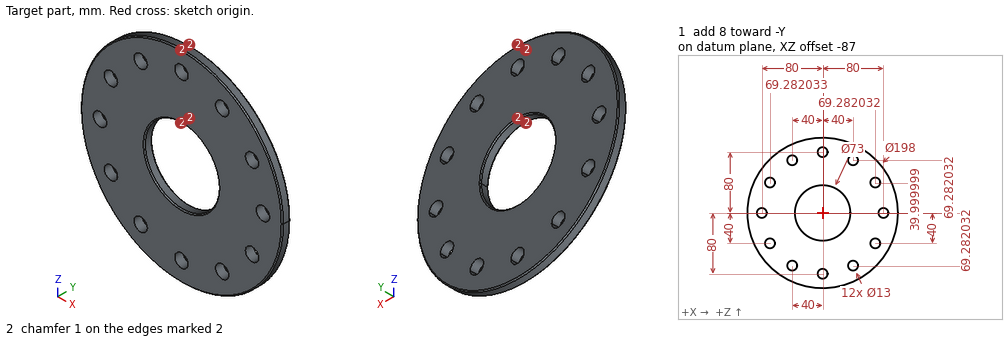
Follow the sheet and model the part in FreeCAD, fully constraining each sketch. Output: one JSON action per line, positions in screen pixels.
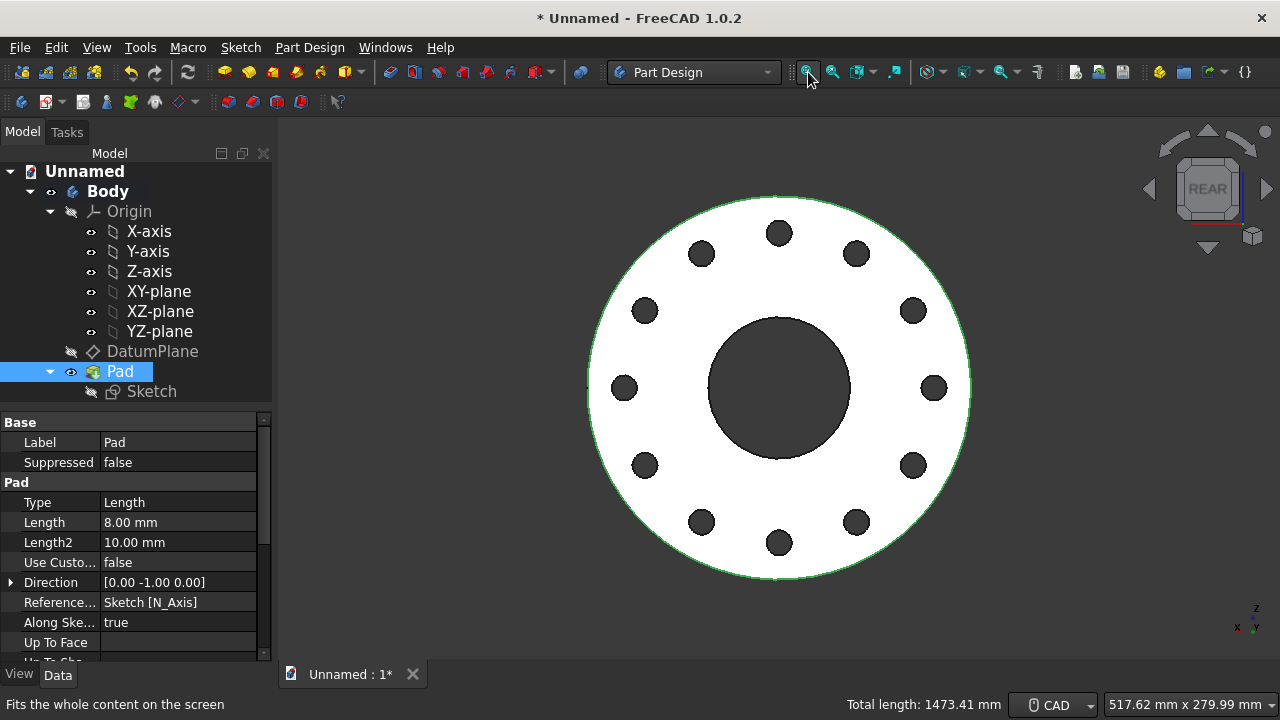
{"action": "left_click", "coordinate": [850, 387], "text": "ctrl"}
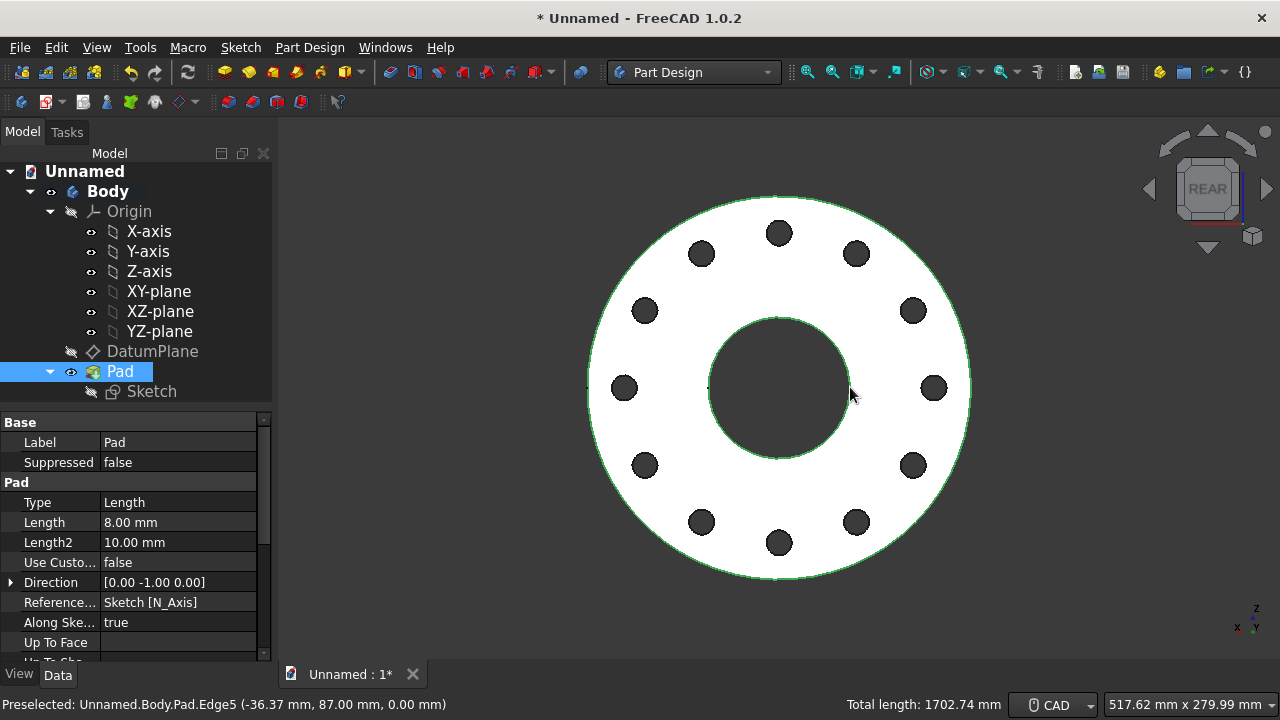
{"action": "left_click", "coordinate": [254, 102]}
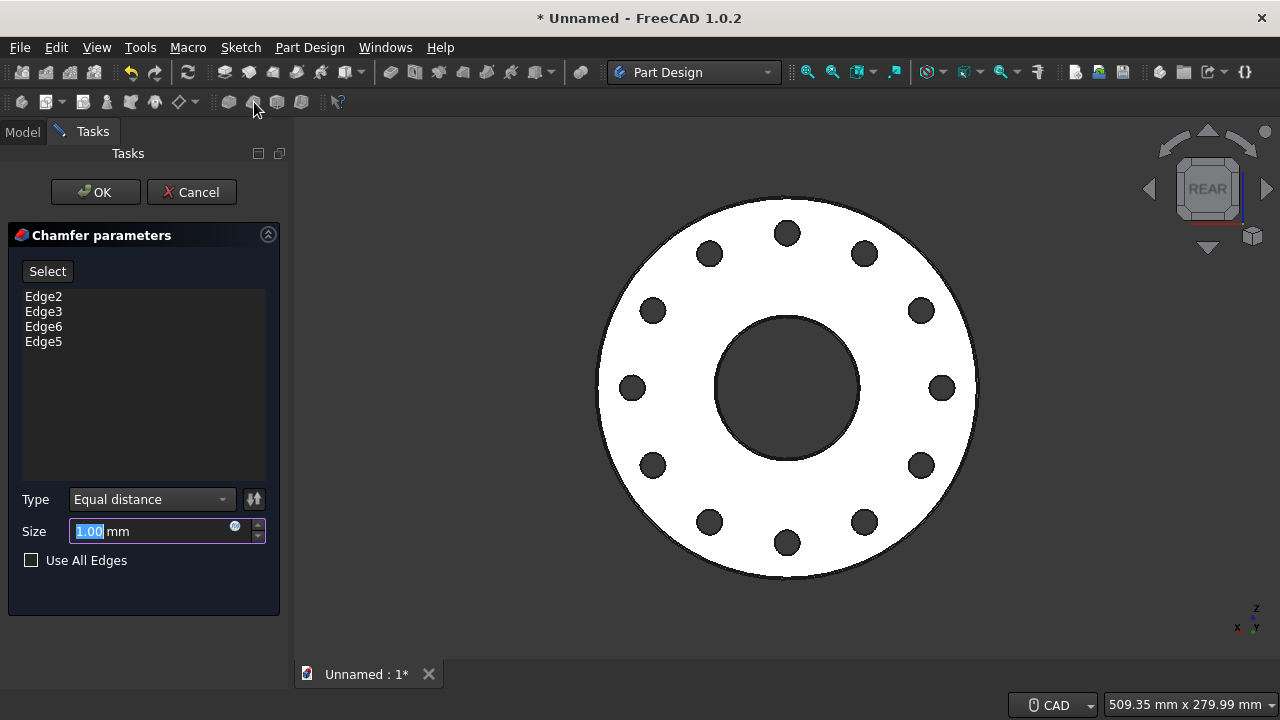
{"action": "type", "text": "1"}
{"action": "key", "text": "Tab"}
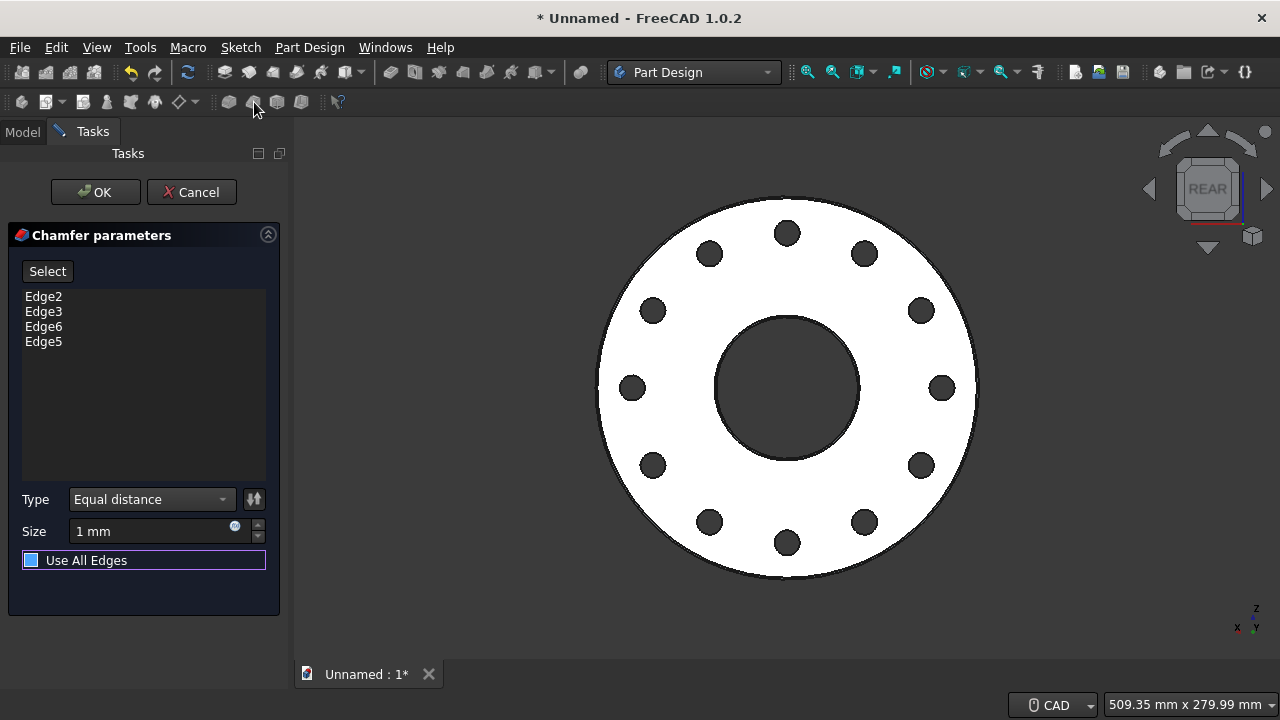
{"action": "left_click", "coordinate": [96, 192]}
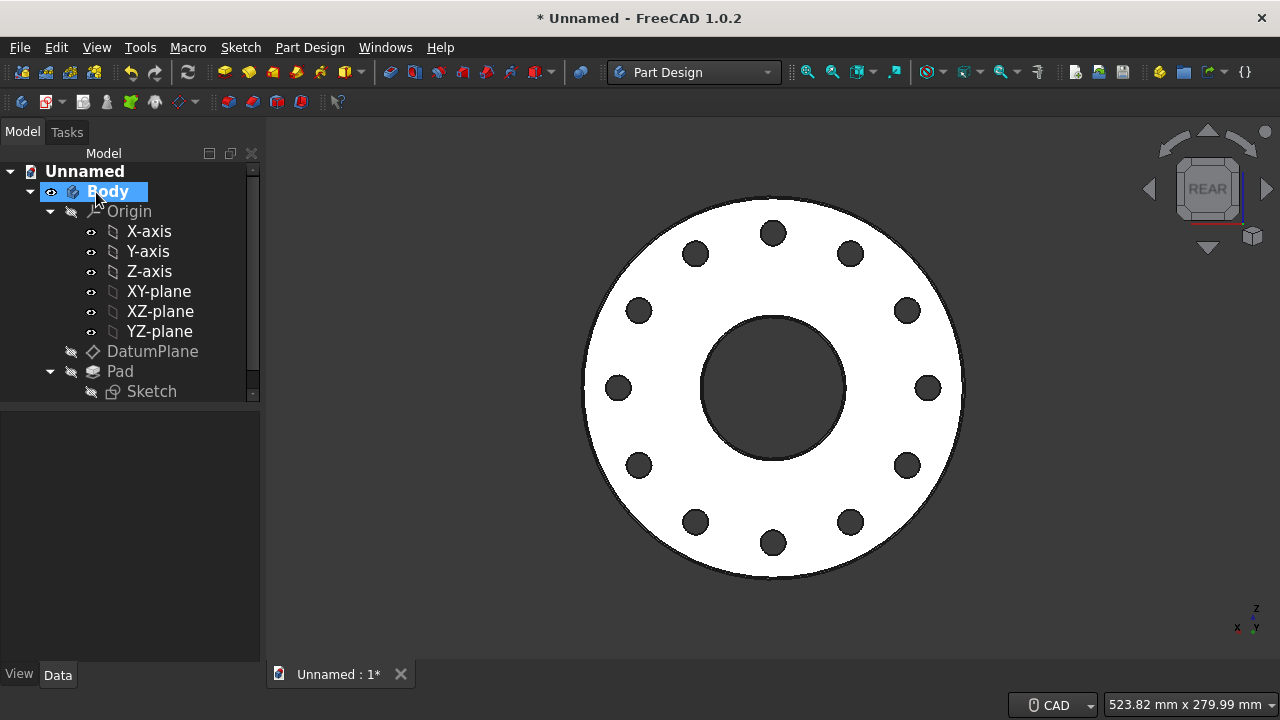
{"action": "key", "text": "0"}